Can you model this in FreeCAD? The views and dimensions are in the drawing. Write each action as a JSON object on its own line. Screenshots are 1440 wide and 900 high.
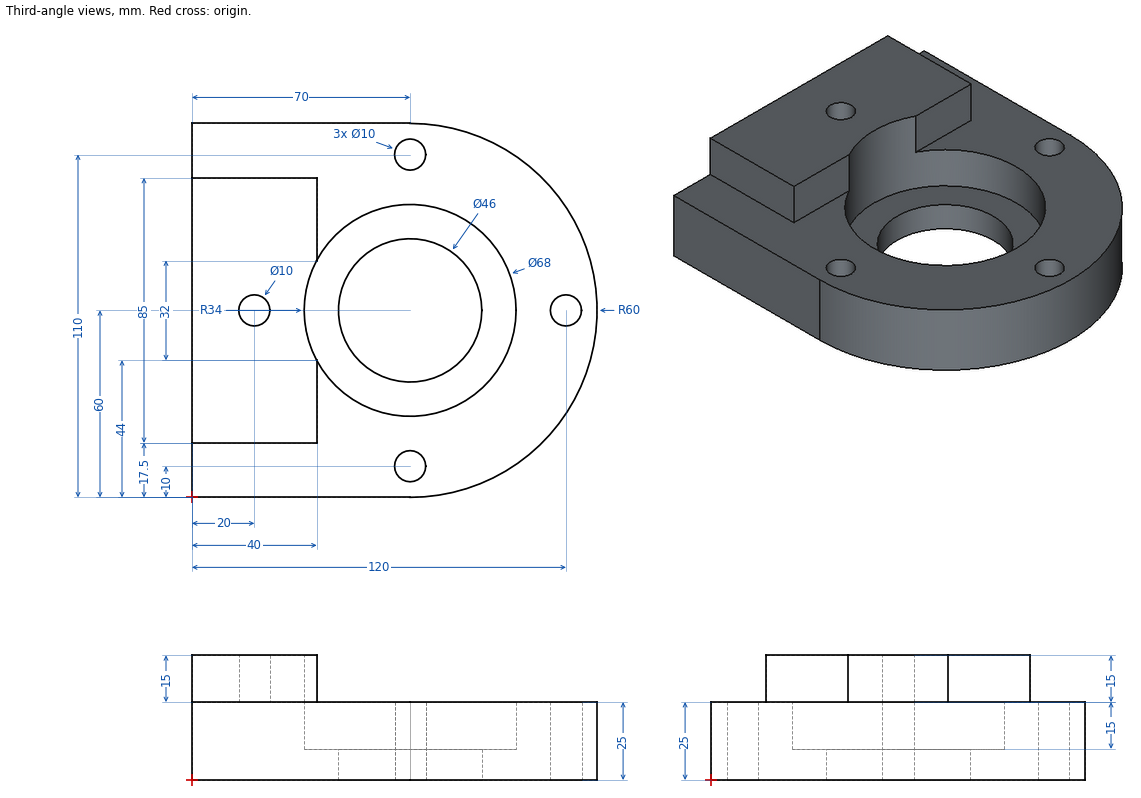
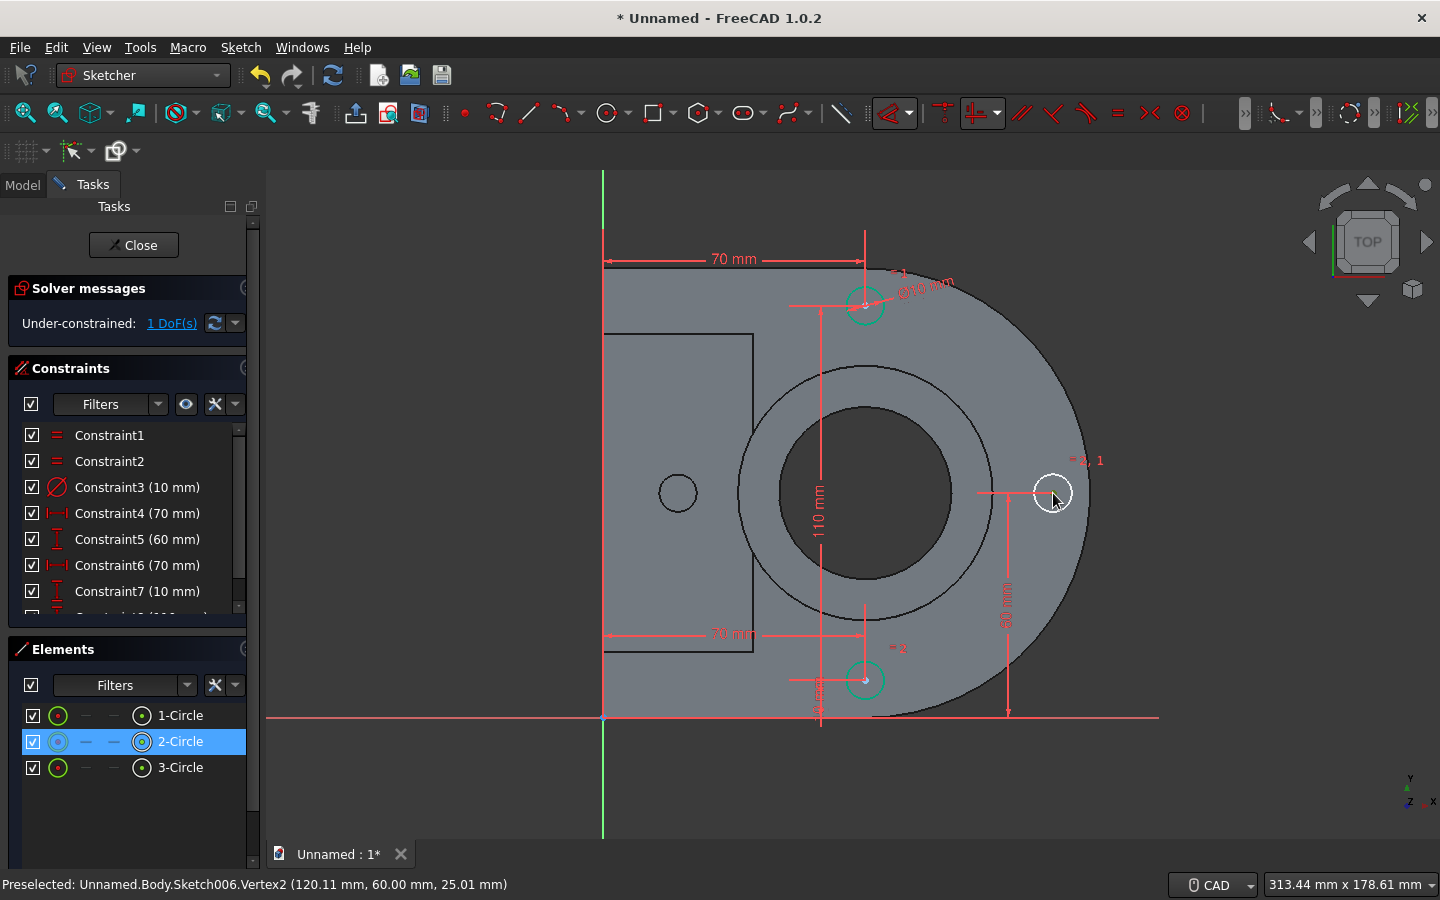
{"action": "key", "text": "l"}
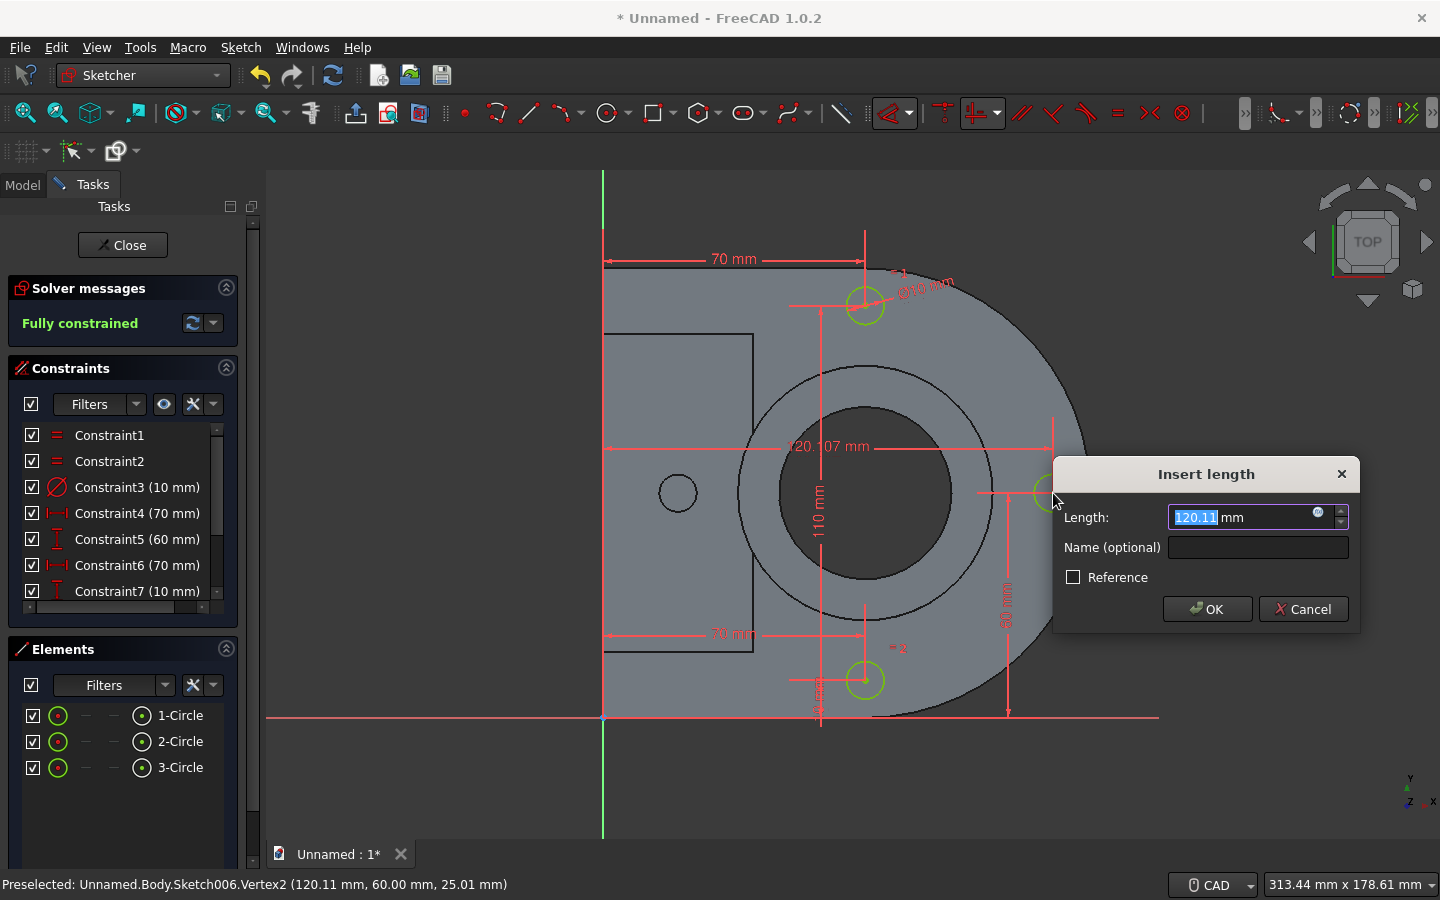
{"action": "type", "text": "120"}
{"action": "key", "text": "Return"}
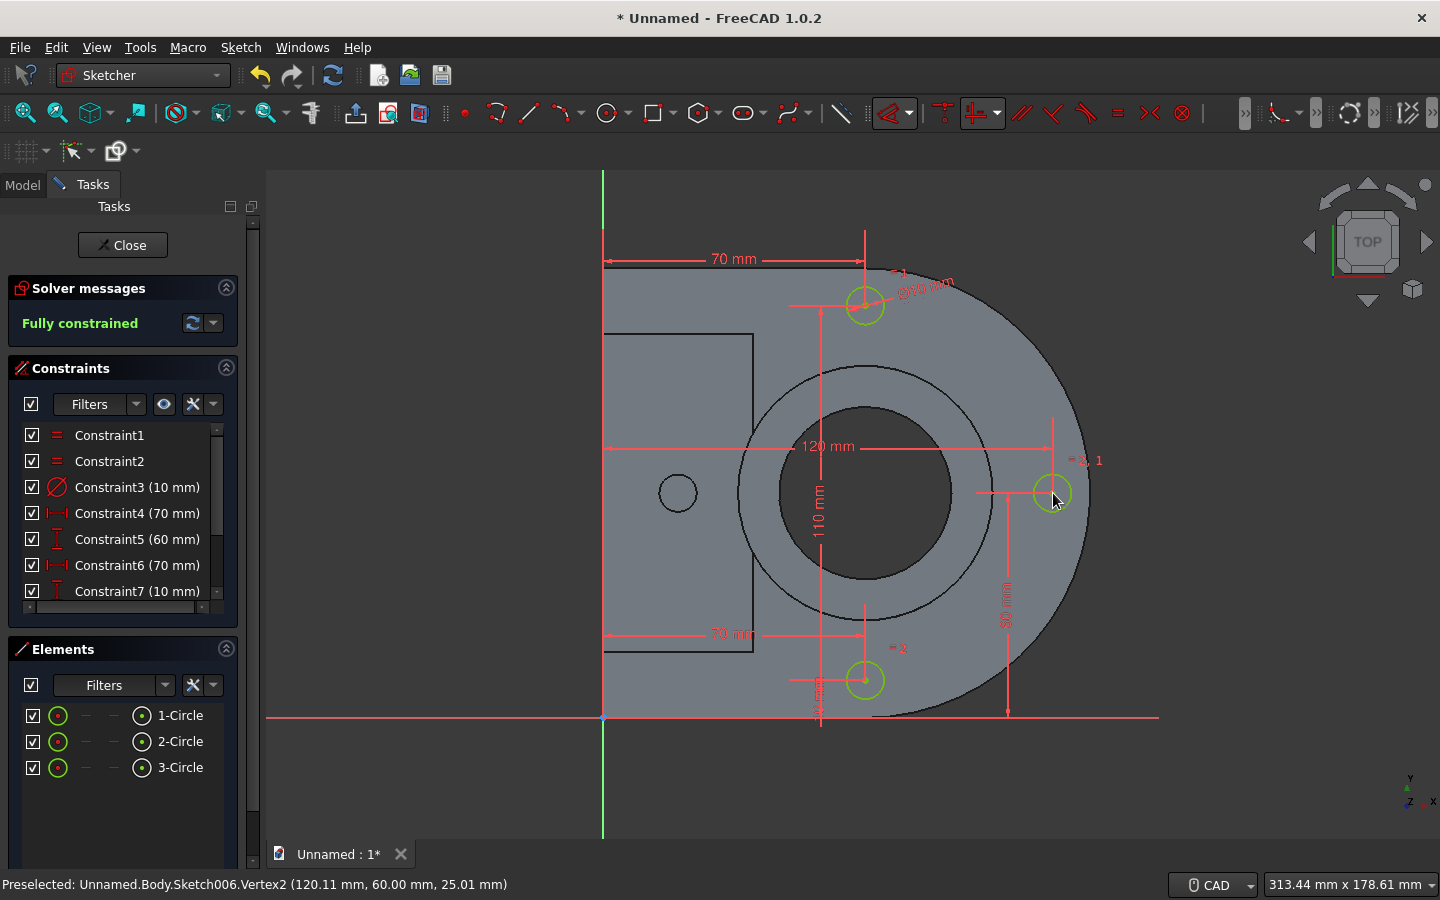
{"action": "left_click", "coordinate": [123, 245]}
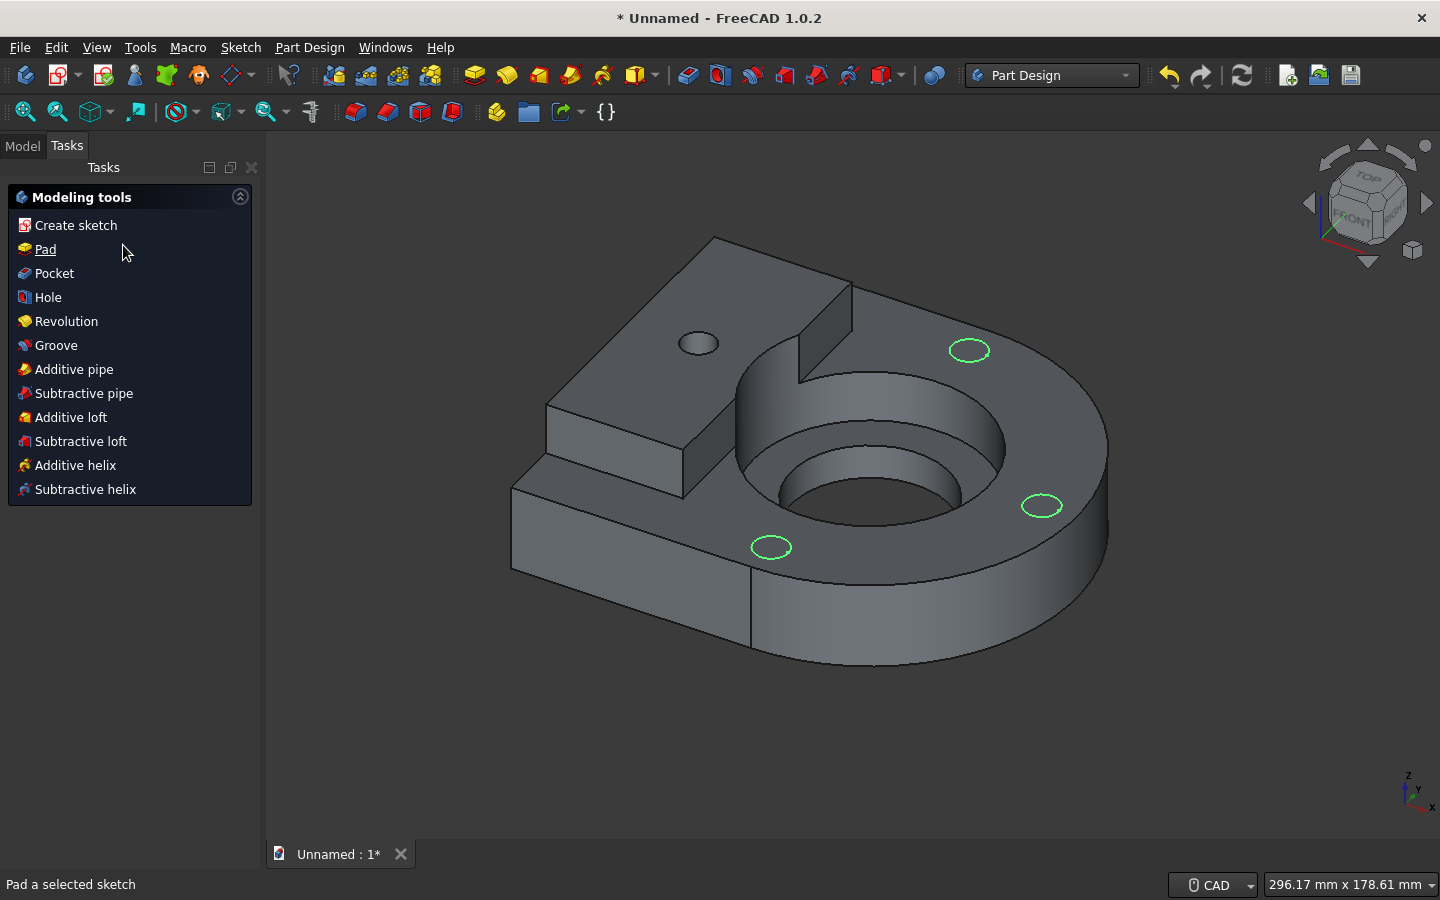
{"action": "left_click", "coordinate": [690, 76]}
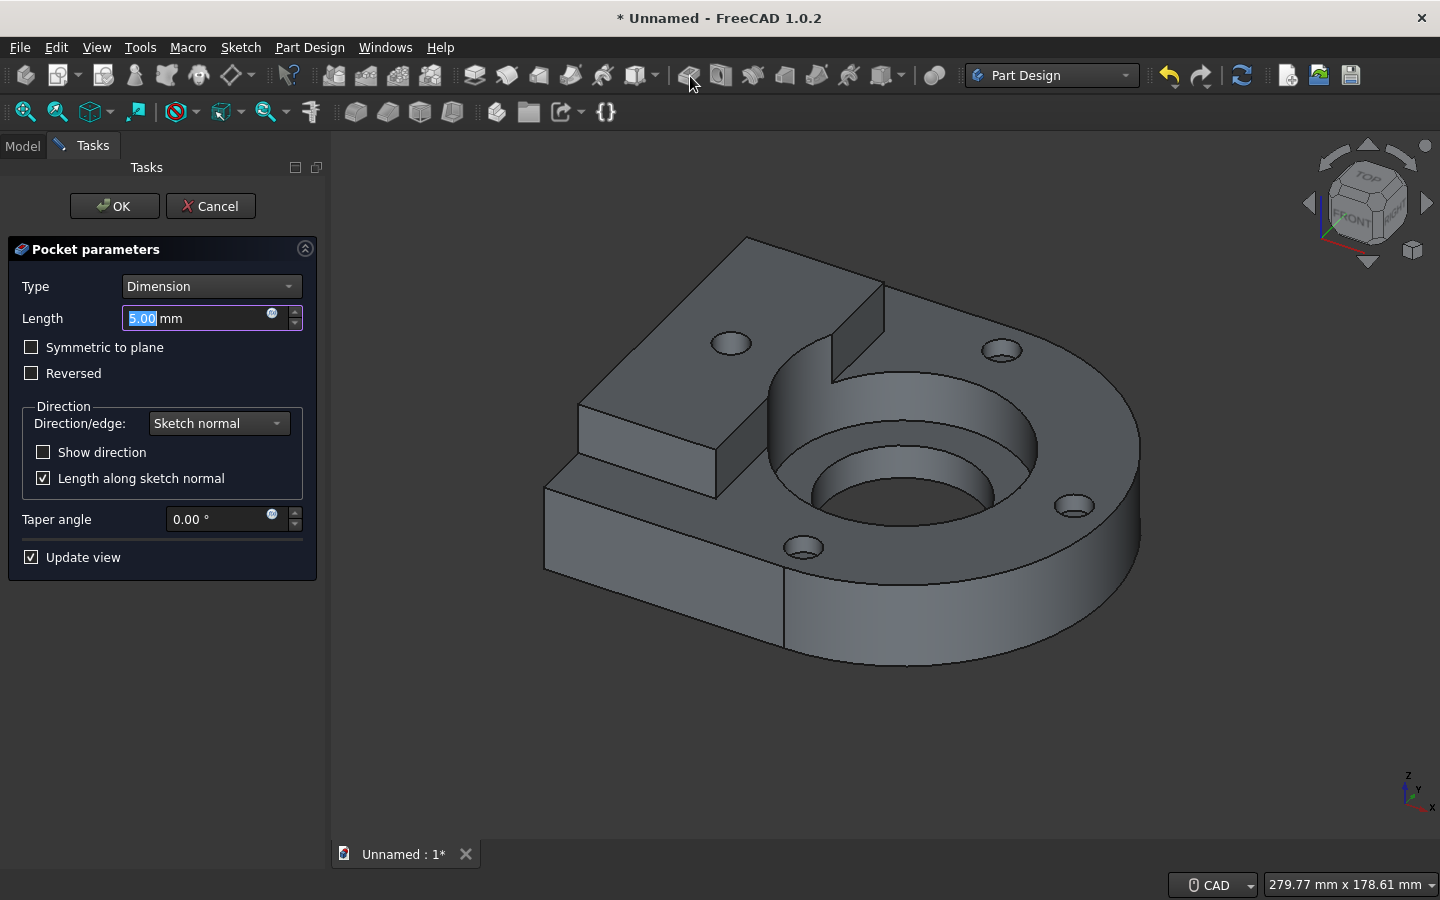
{"action": "type", "text": "25"}
{"action": "key", "text": "Tab"}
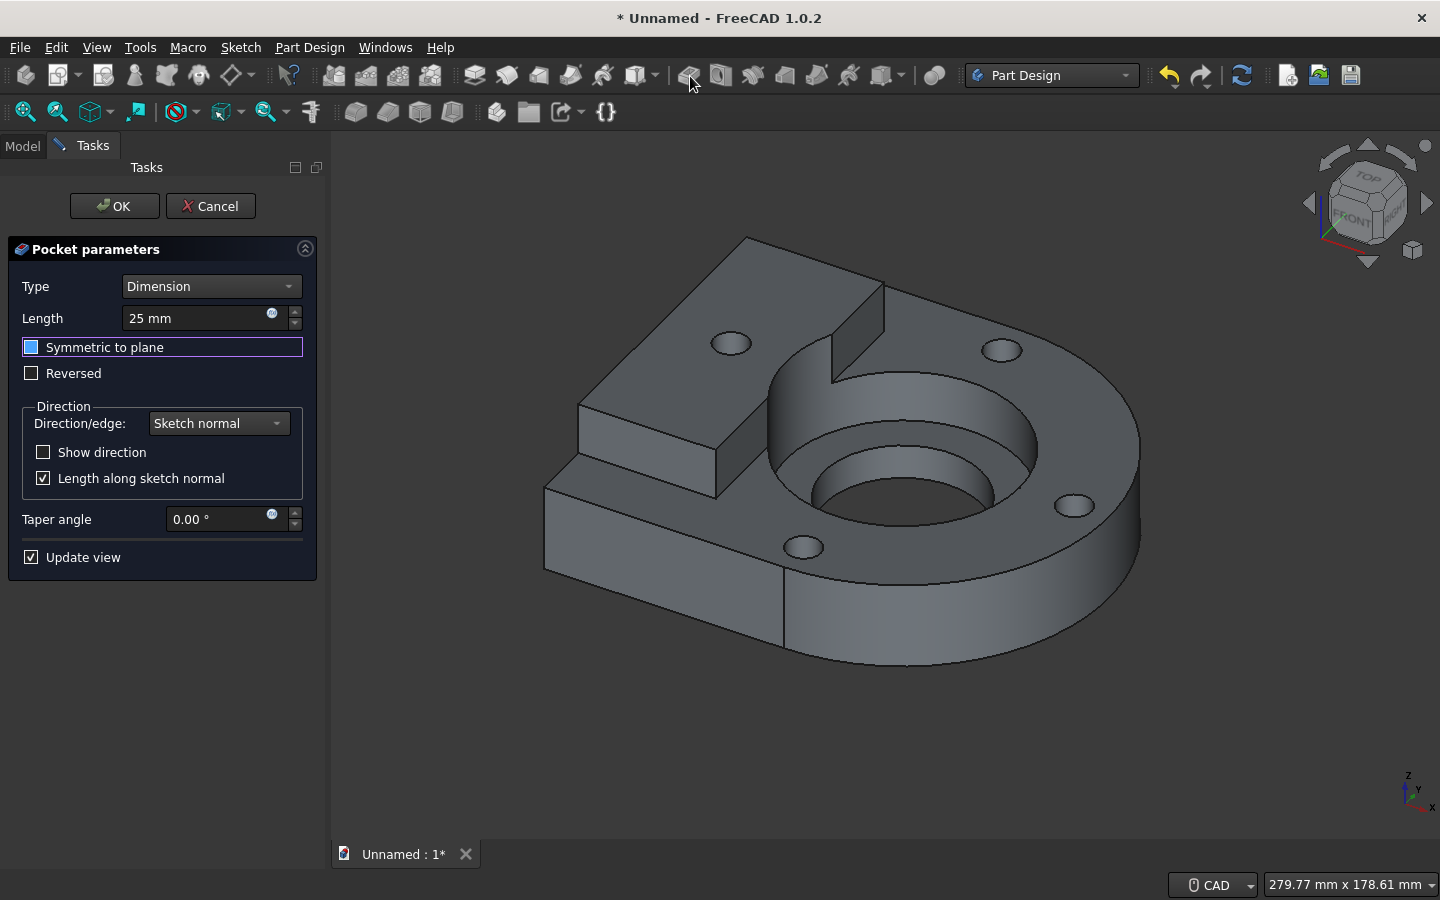
{"action": "left_click", "coordinate": [115, 206]}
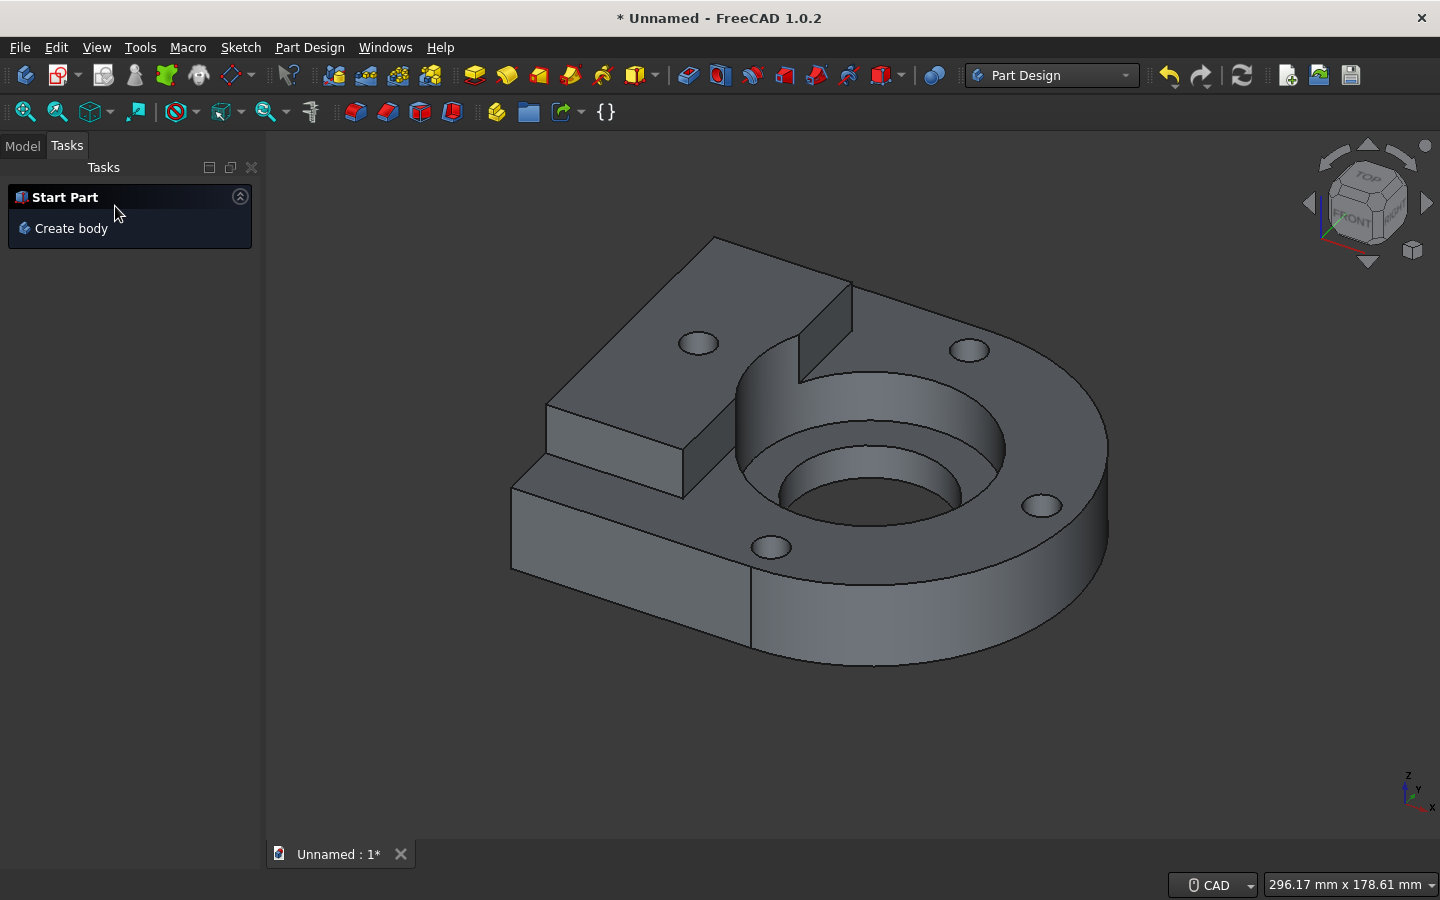
{"action": "key", "text": "0"}